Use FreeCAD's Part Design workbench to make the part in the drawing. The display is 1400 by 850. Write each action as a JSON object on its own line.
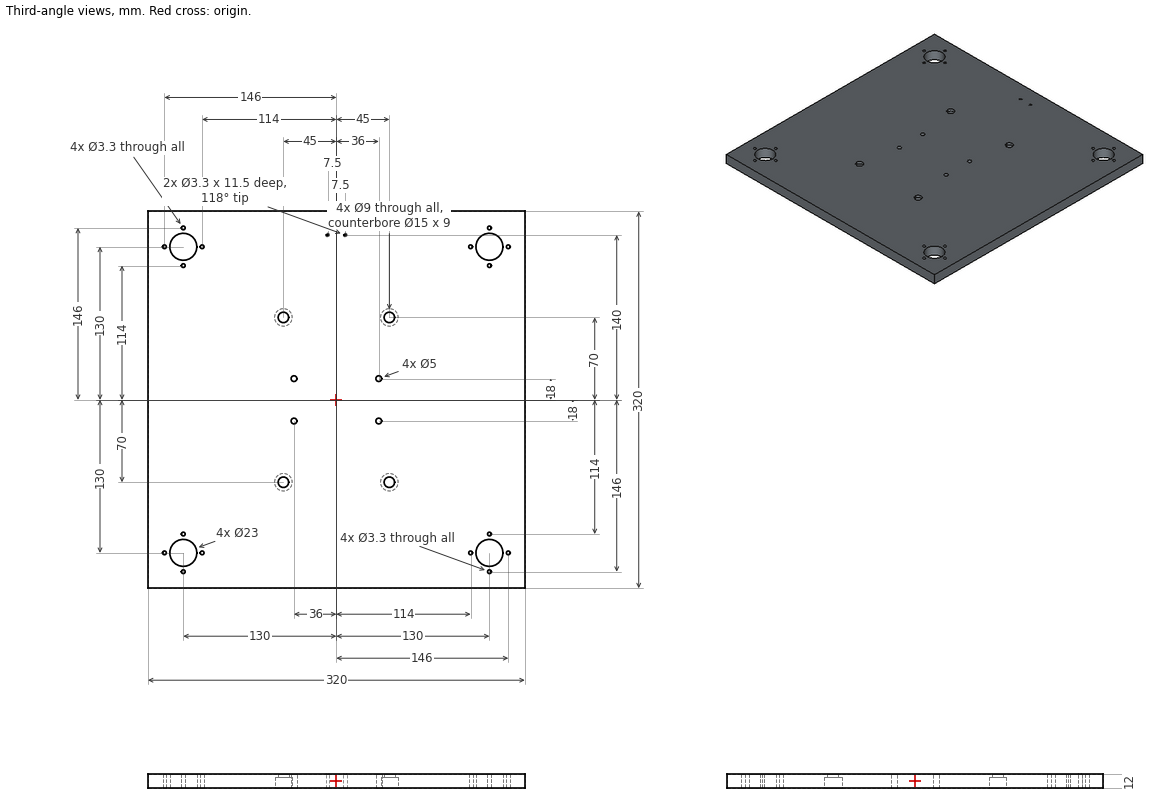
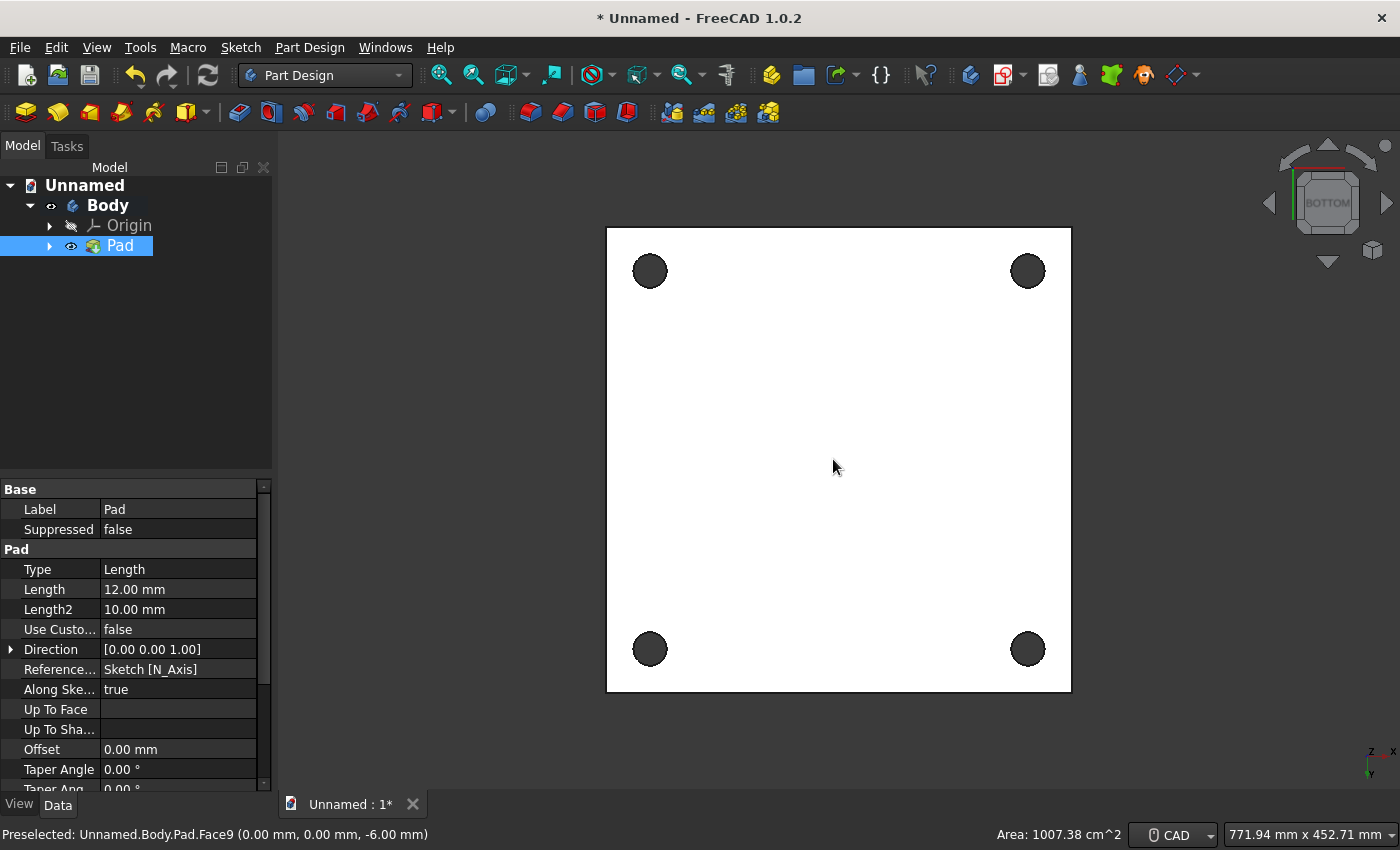
{"action": "left_click", "coordinate": [1004, 76]}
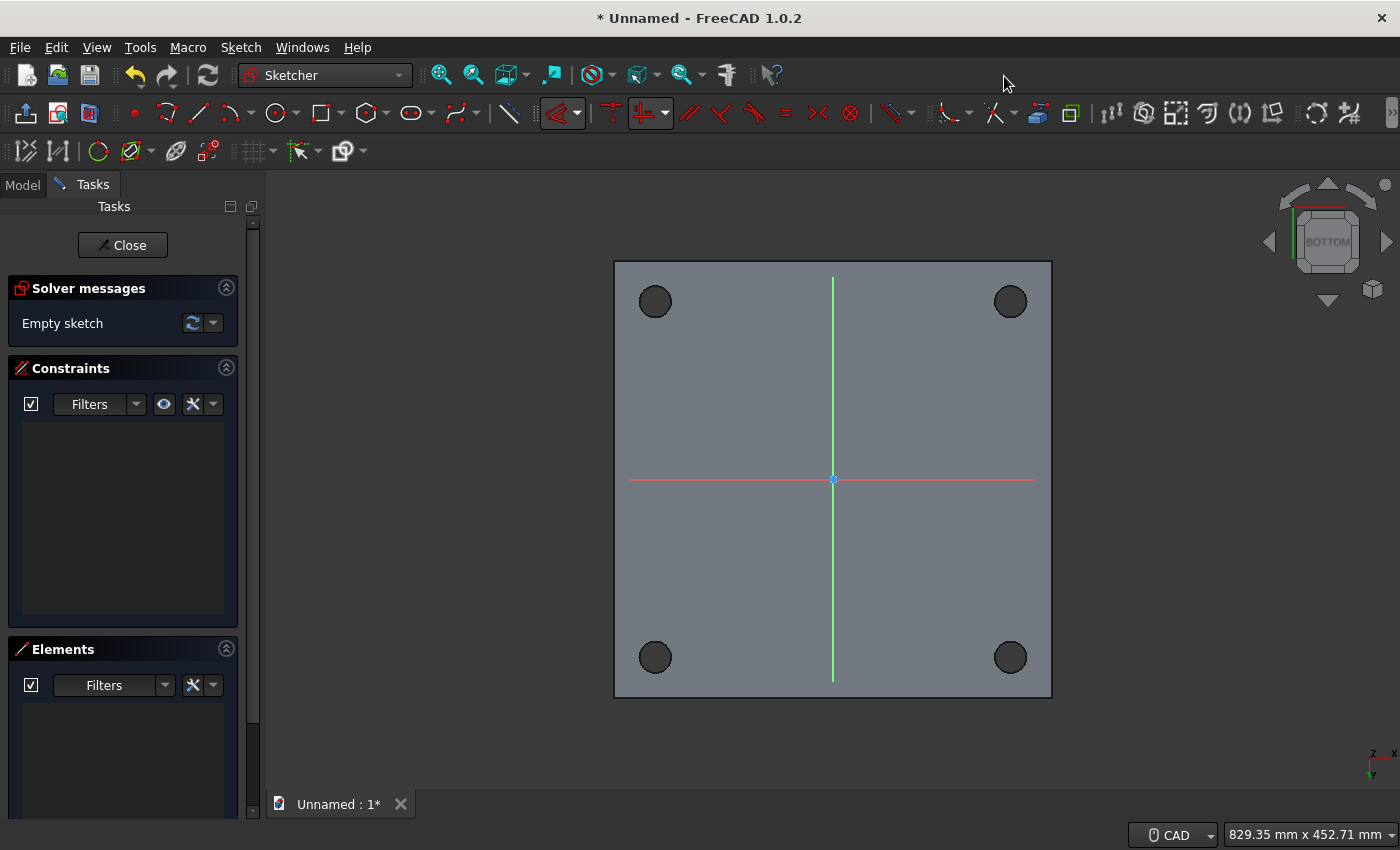
{"action": "scroll", "coordinate": [847, 480], "scroll_direction": "up", "scroll_amount": 9}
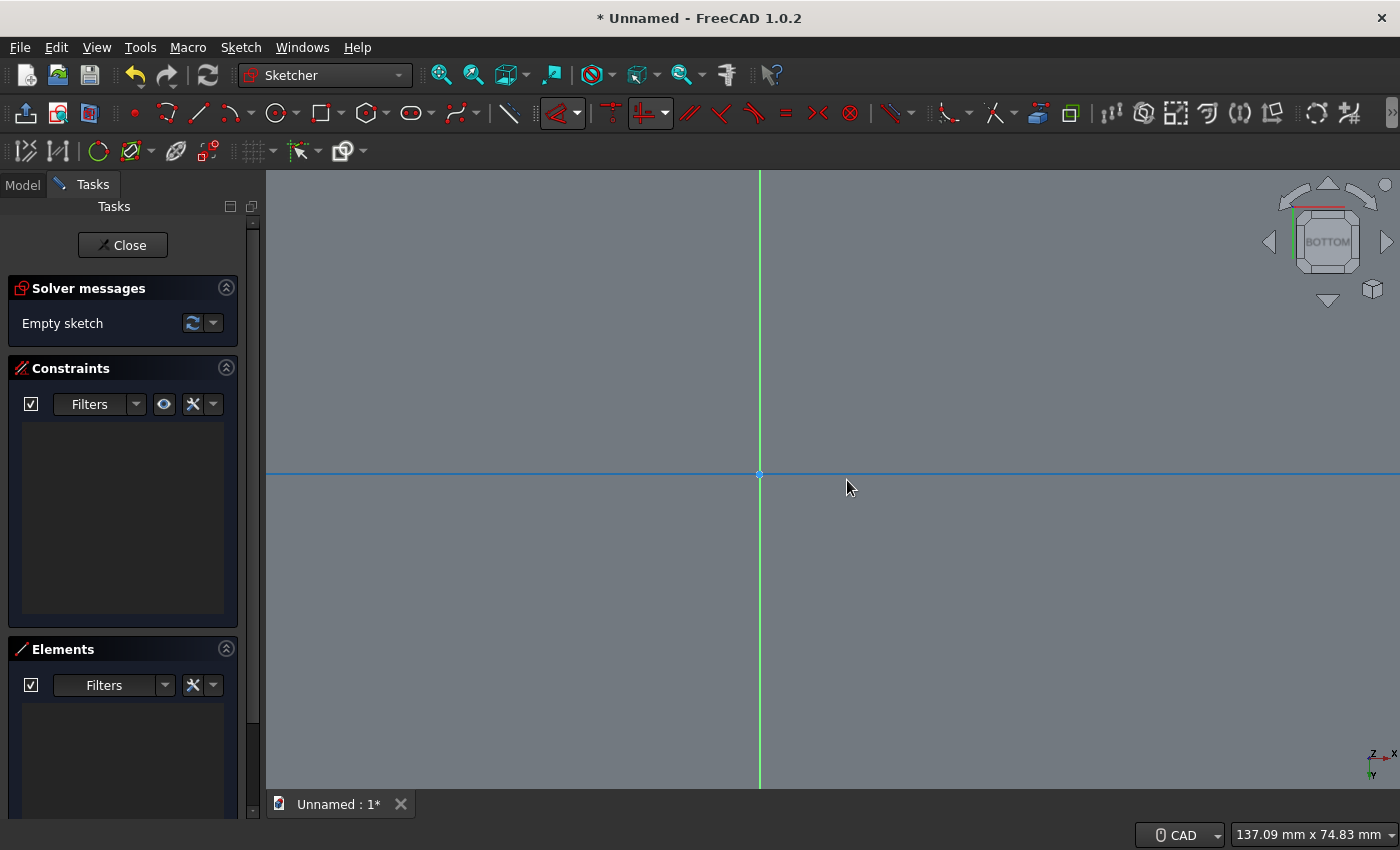
{"action": "left_click", "coordinate": [276, 114]}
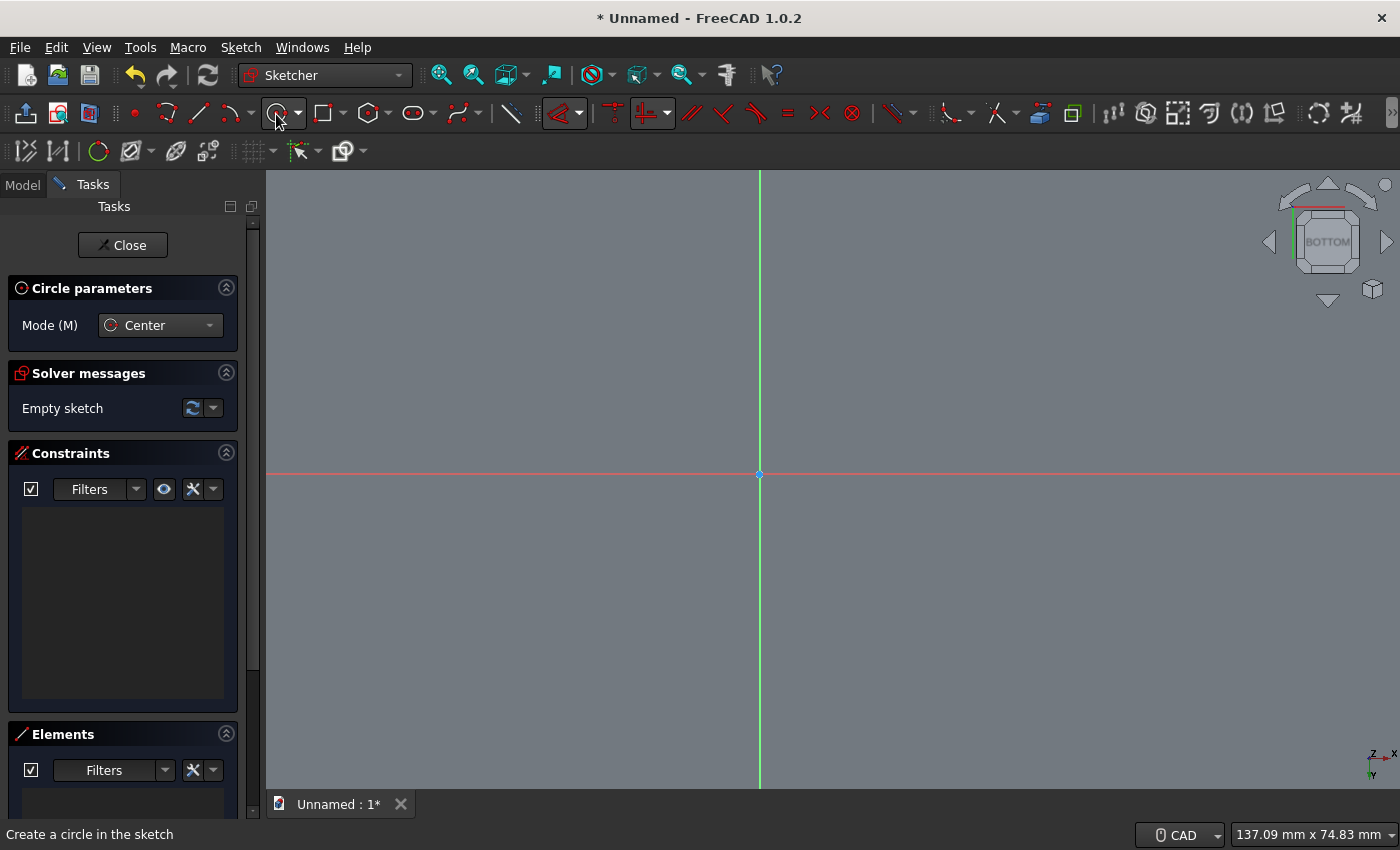
{"action": "left_click", "coordinate": [1058, 623]}
{"action": "mouse_move", "coordinate": [1072, 609]}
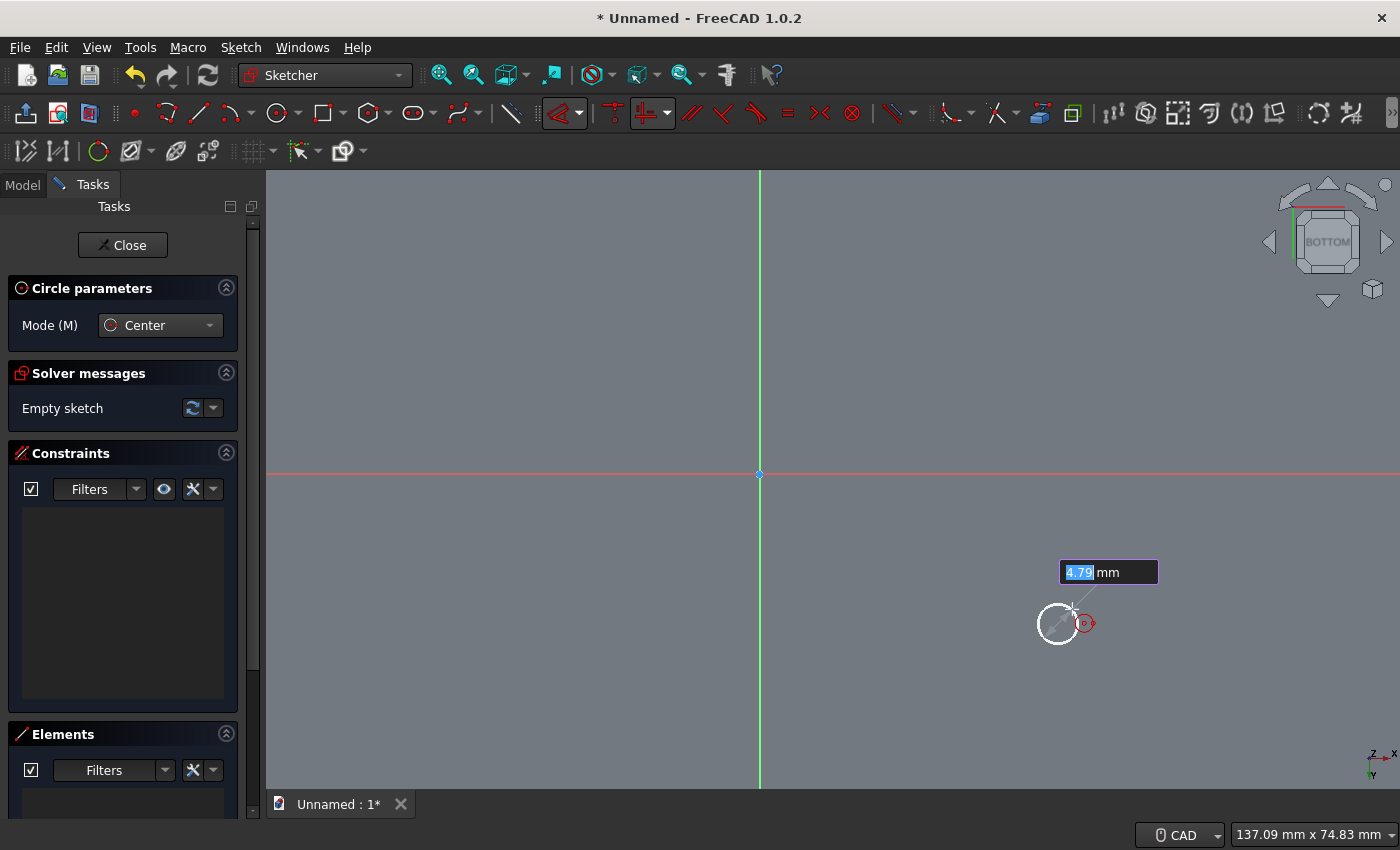
{"action": "type", "text": "5"}
{"action": "key", "text": "Return"}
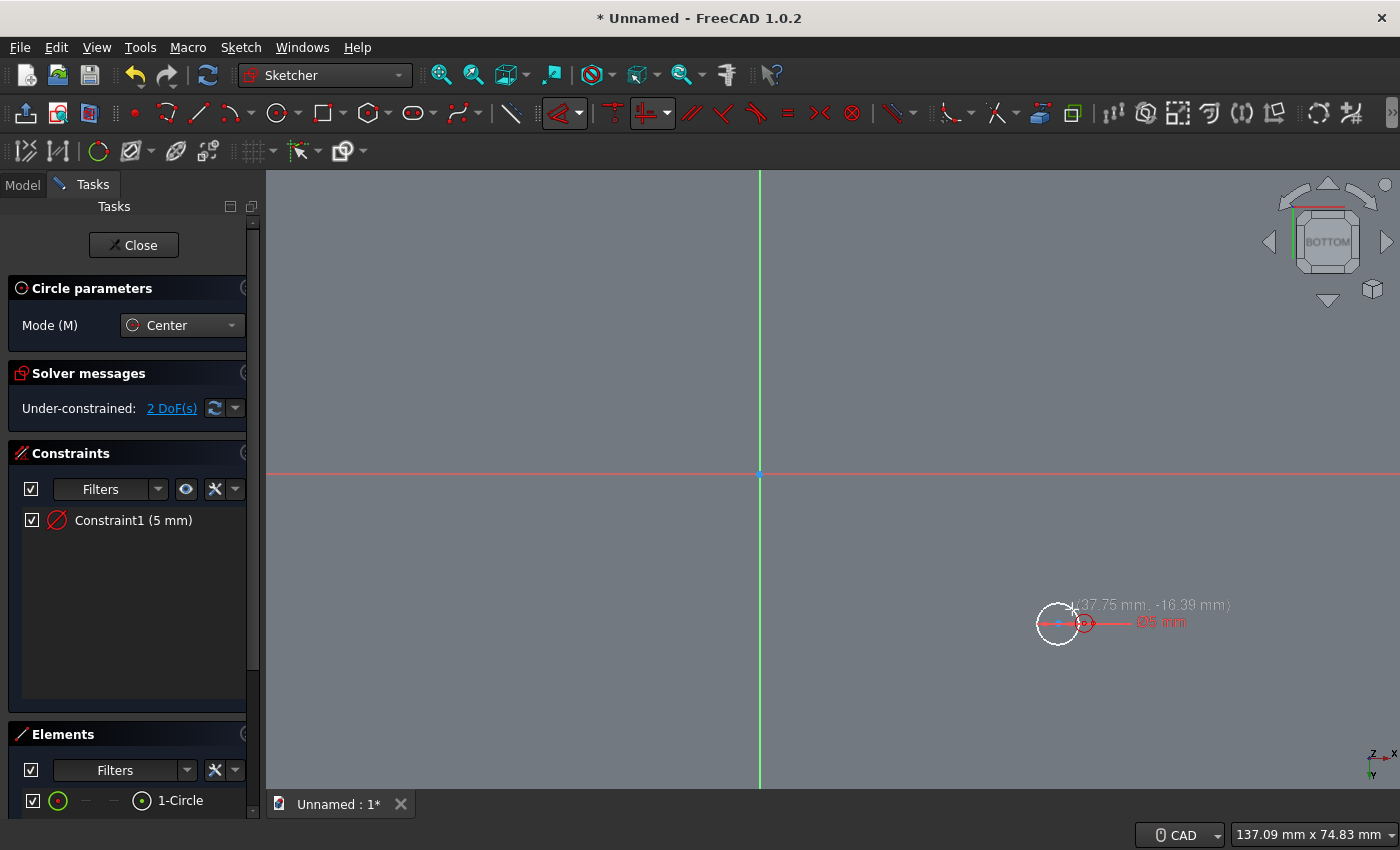
{"action": "left_click", "coordinate": [1058, 326]}
{"action": "mouse_move", "coordinate": [1072, 311]}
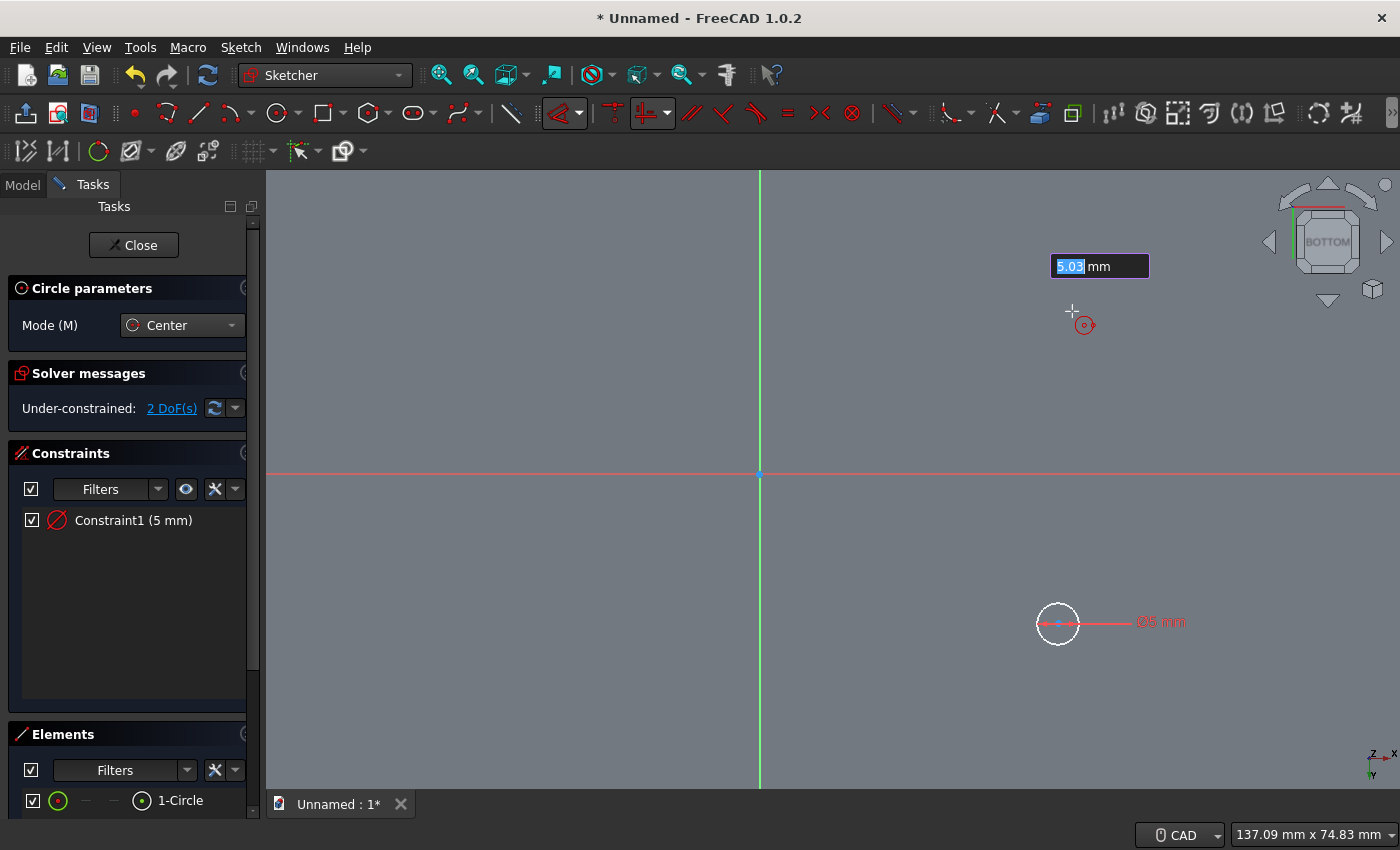
{"action": "type", "text": "5"}
{"action": "key", "text": "Return"}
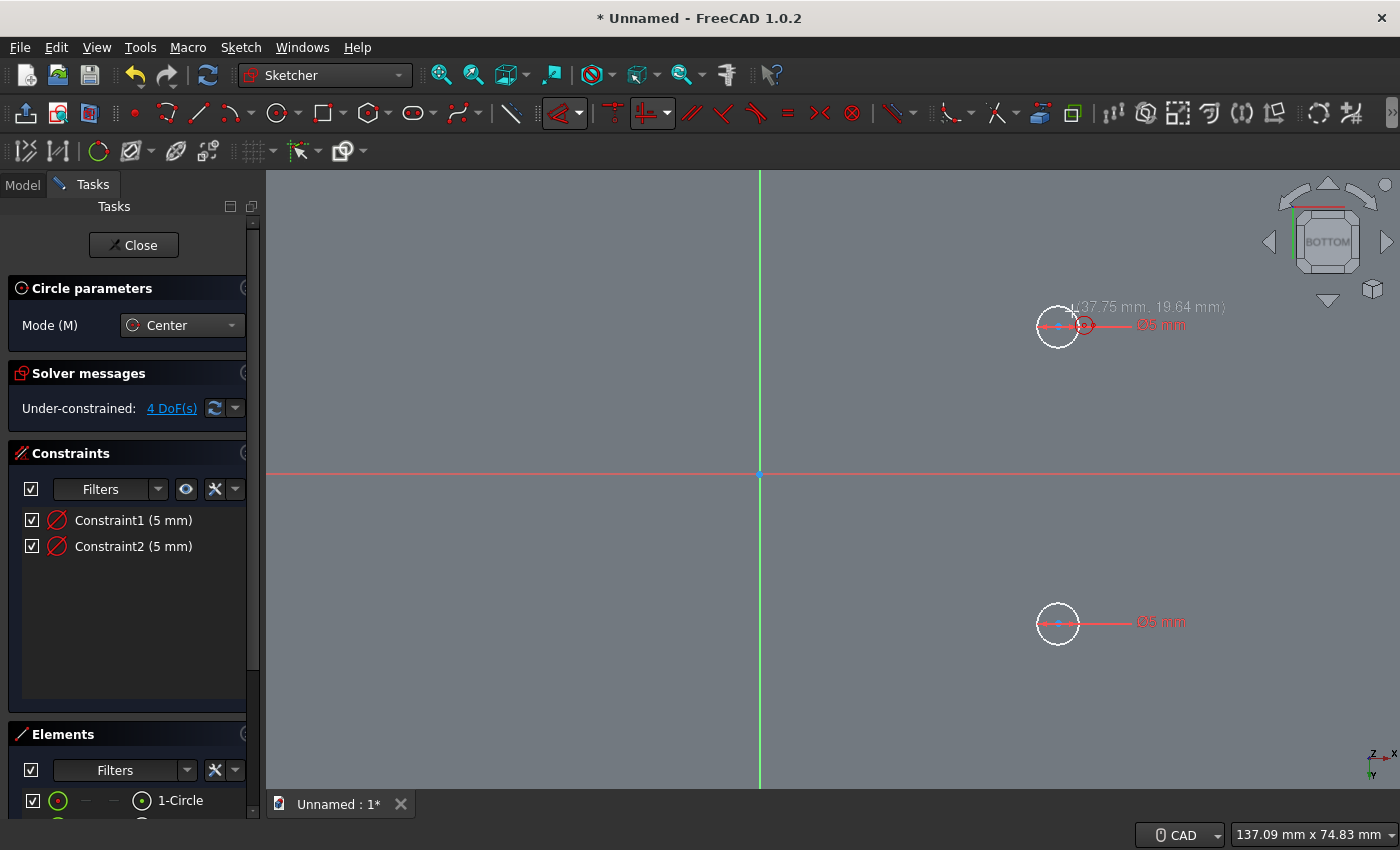
{"action": "left_click", "coordinate": [462, 326]}
{"action": "mouse_move", "coordinate": [477, 311]}